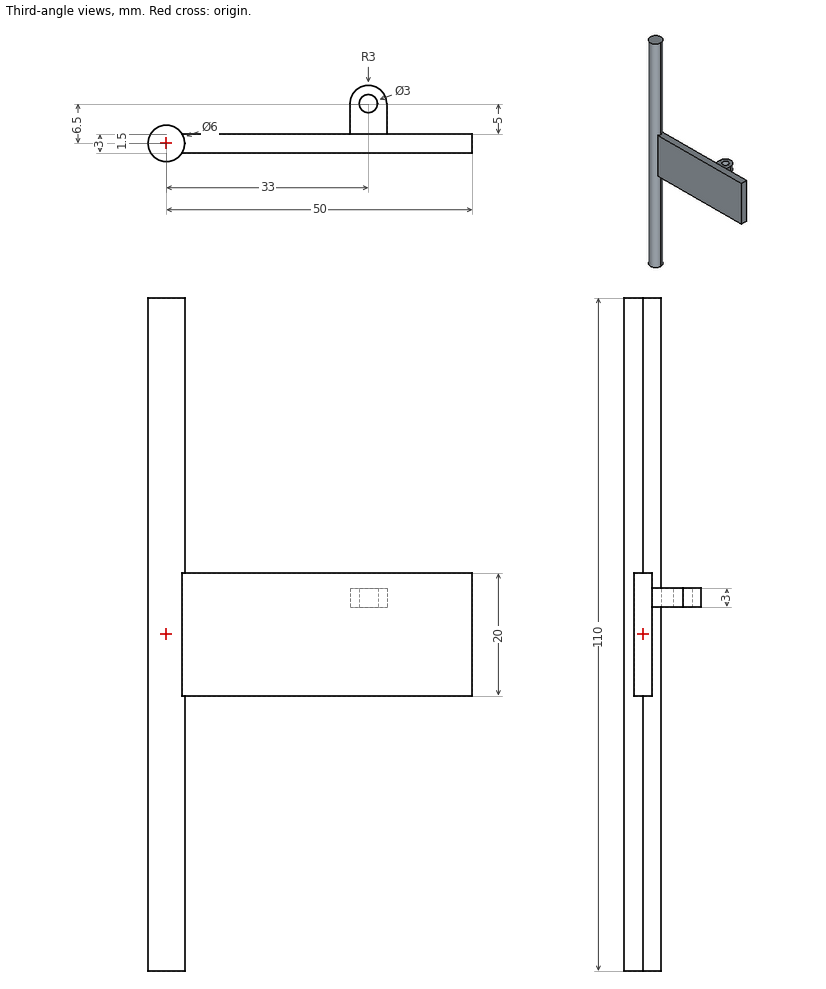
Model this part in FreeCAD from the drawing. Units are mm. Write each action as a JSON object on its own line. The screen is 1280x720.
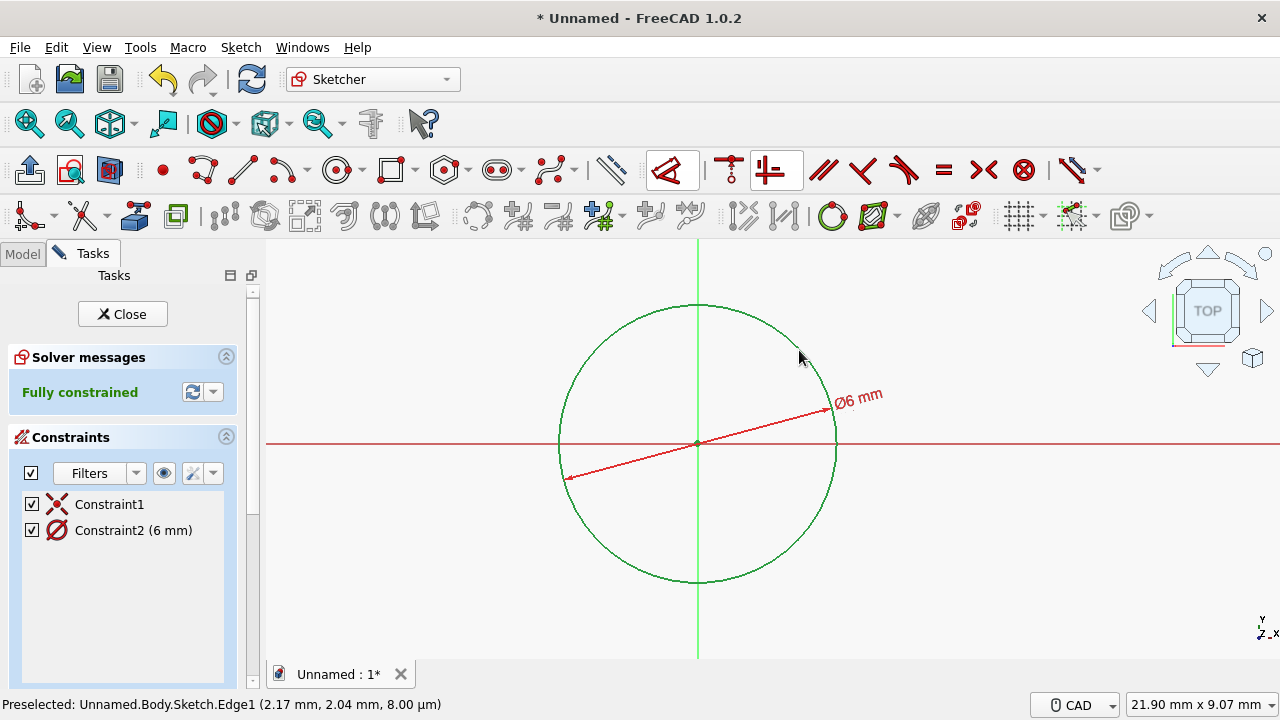
{"action": "left_click", "coordinate": [123, 314]}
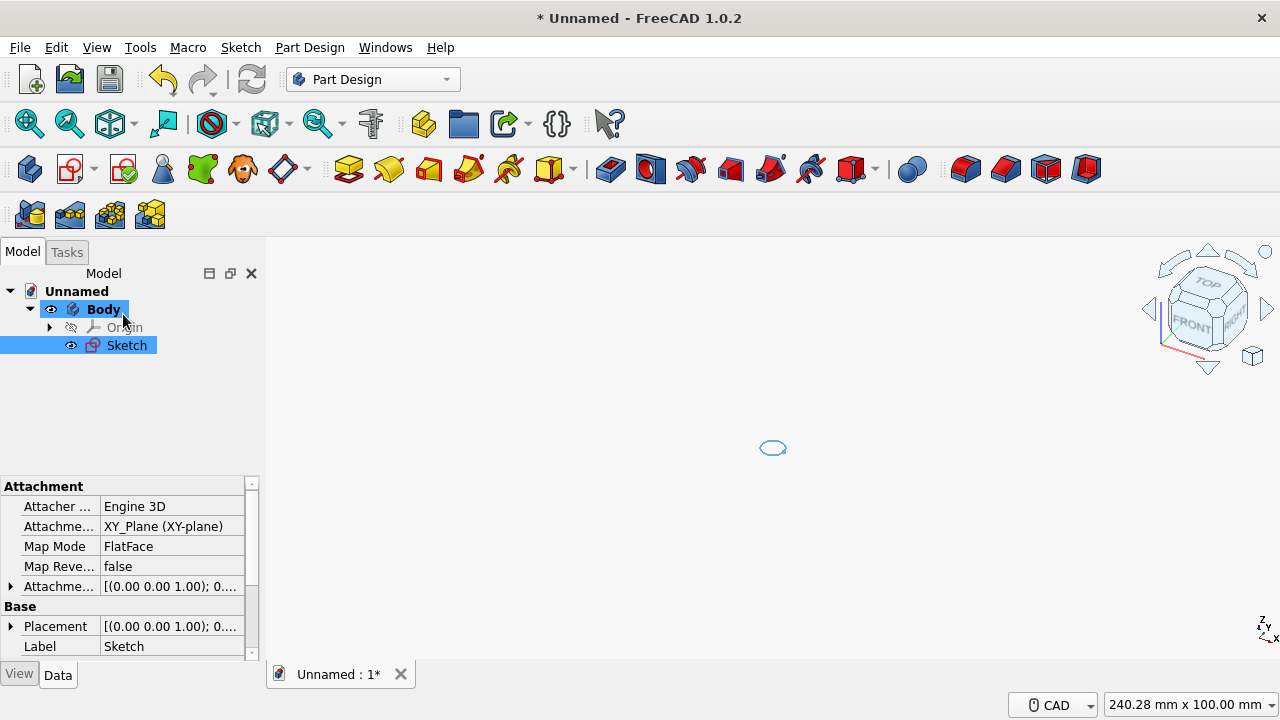
{"action": "left_click", "coordinate": [350, 170]}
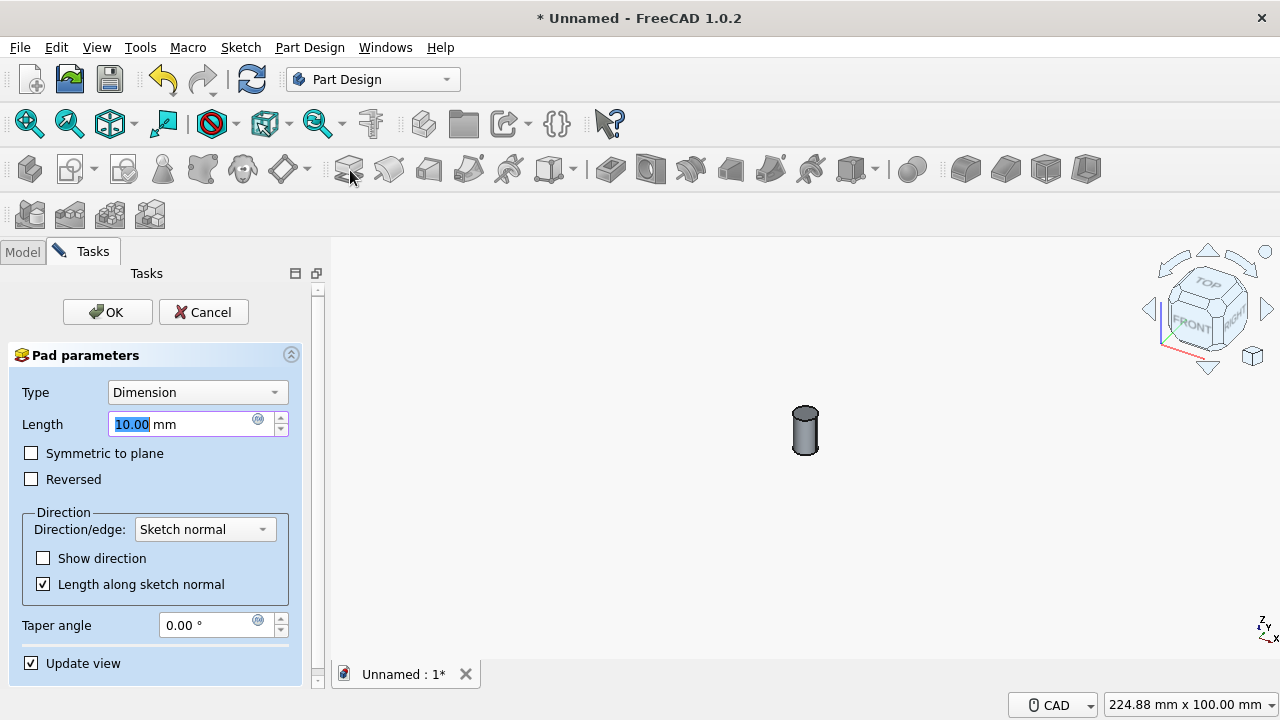
{"action": "type", "text": "110"}
{"action": "key", "text": "Tab"}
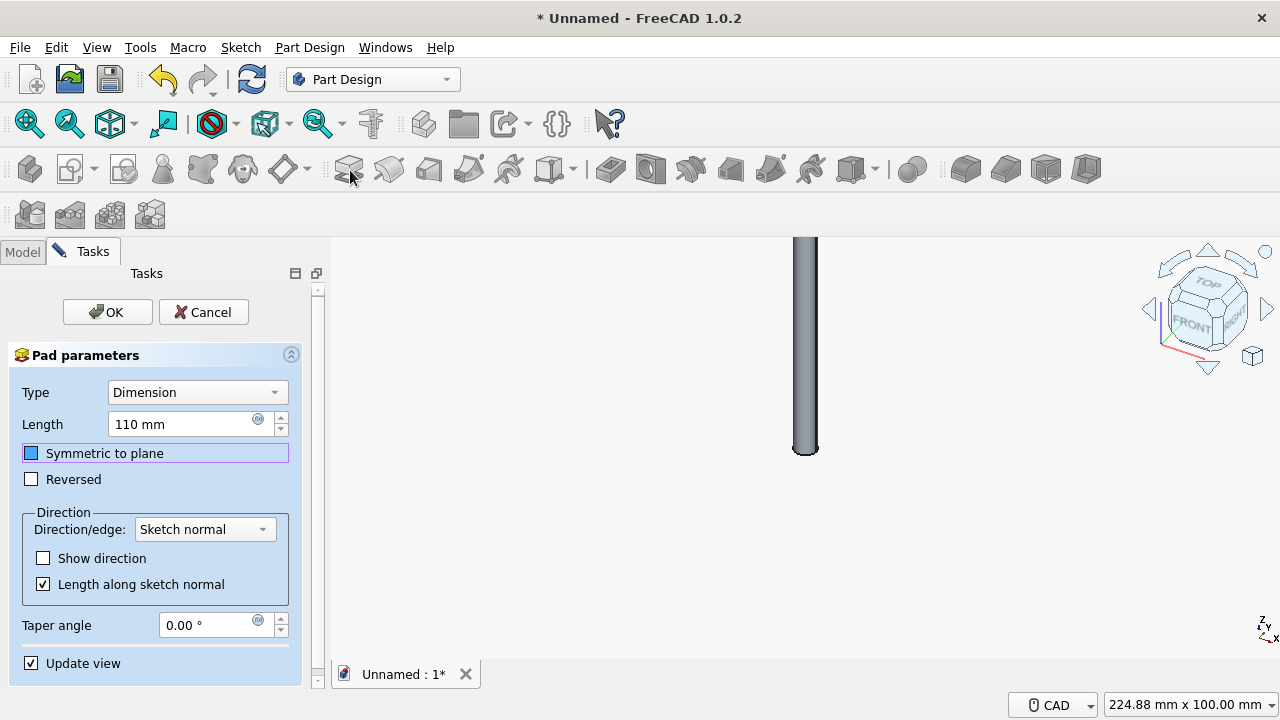
{"action": "left_click", "coordinate": [30, 453]}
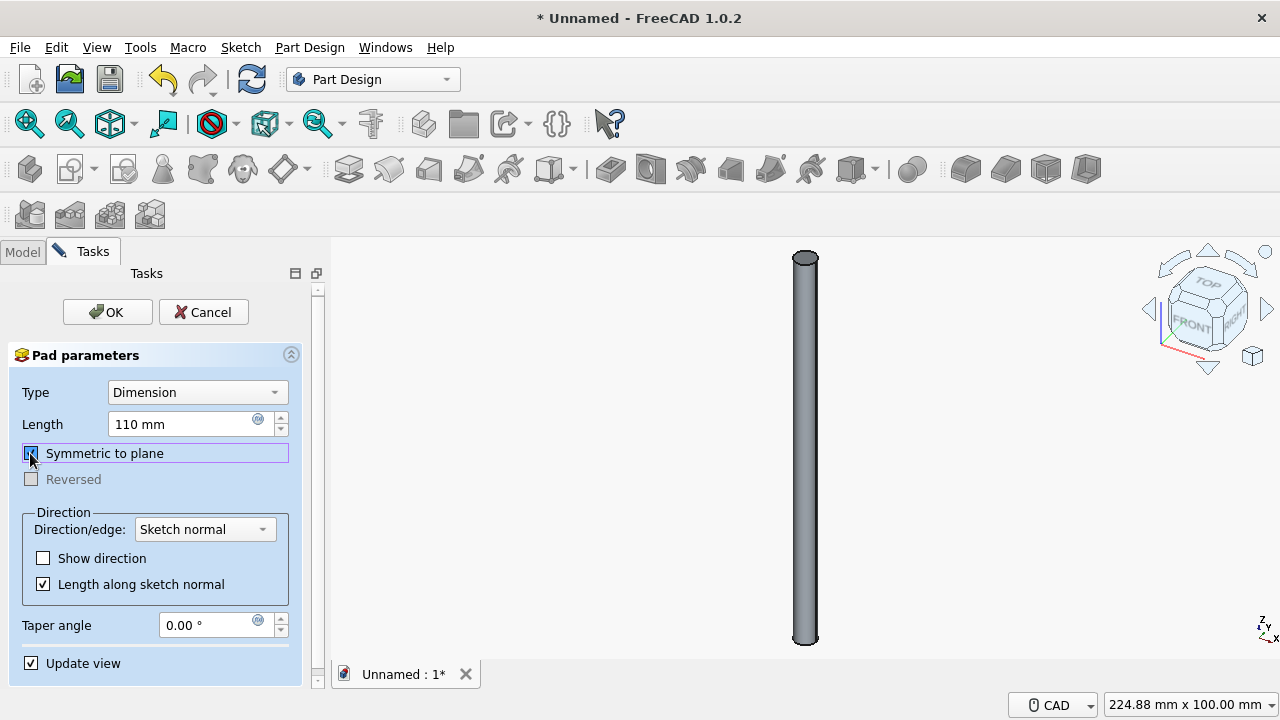
{"action": "left_click", "coordinate": [108, 312]}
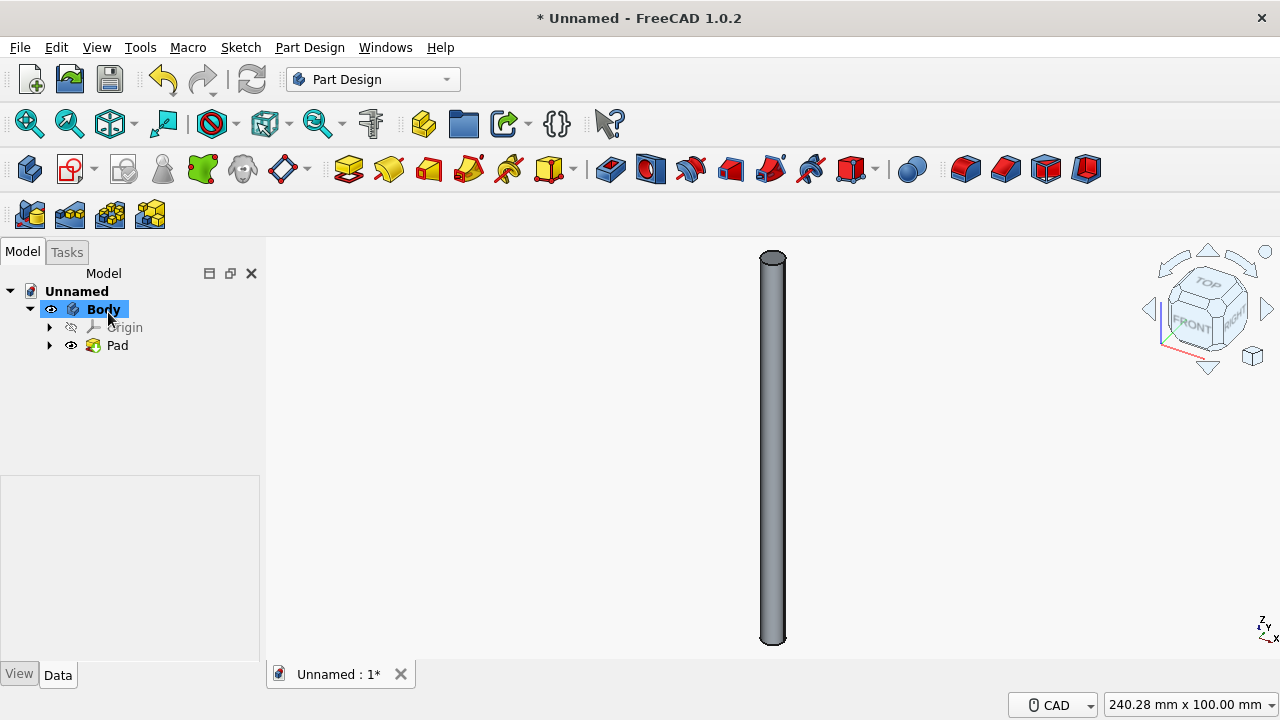
{"action": "left_click", "coordinate": [70, 170]}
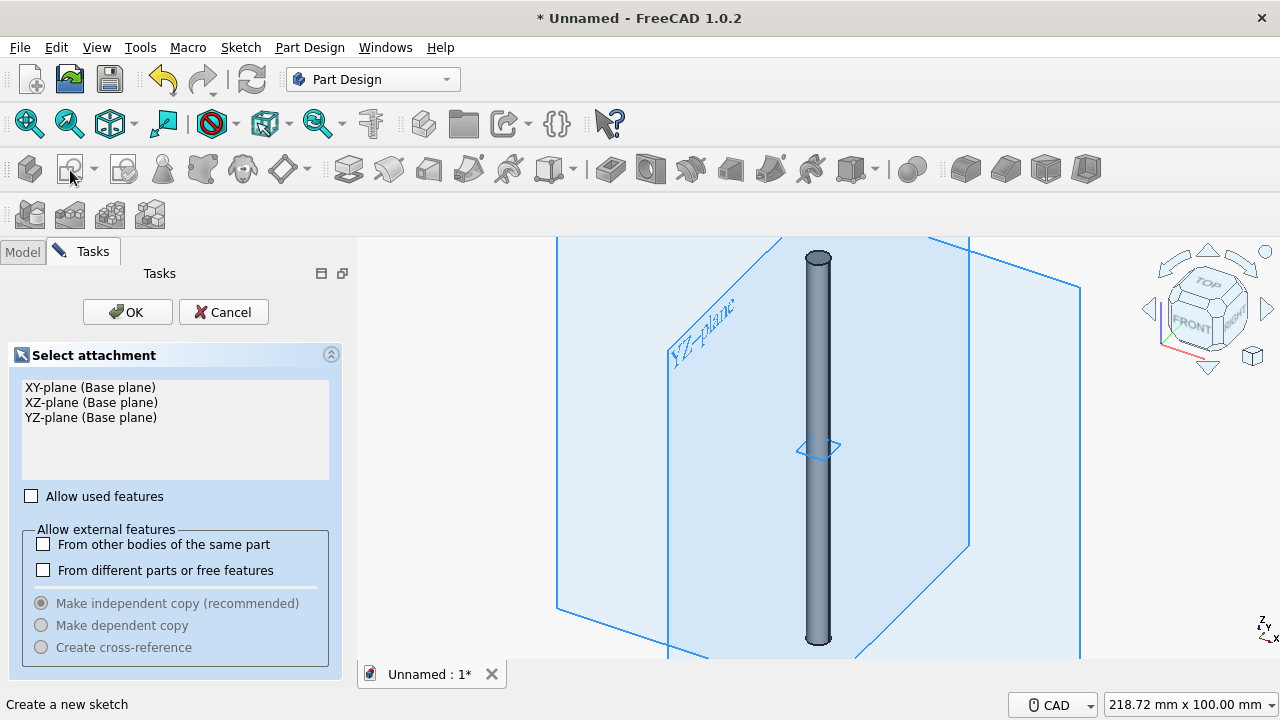
{"action": "left_click", "coordinate": [82, 388]}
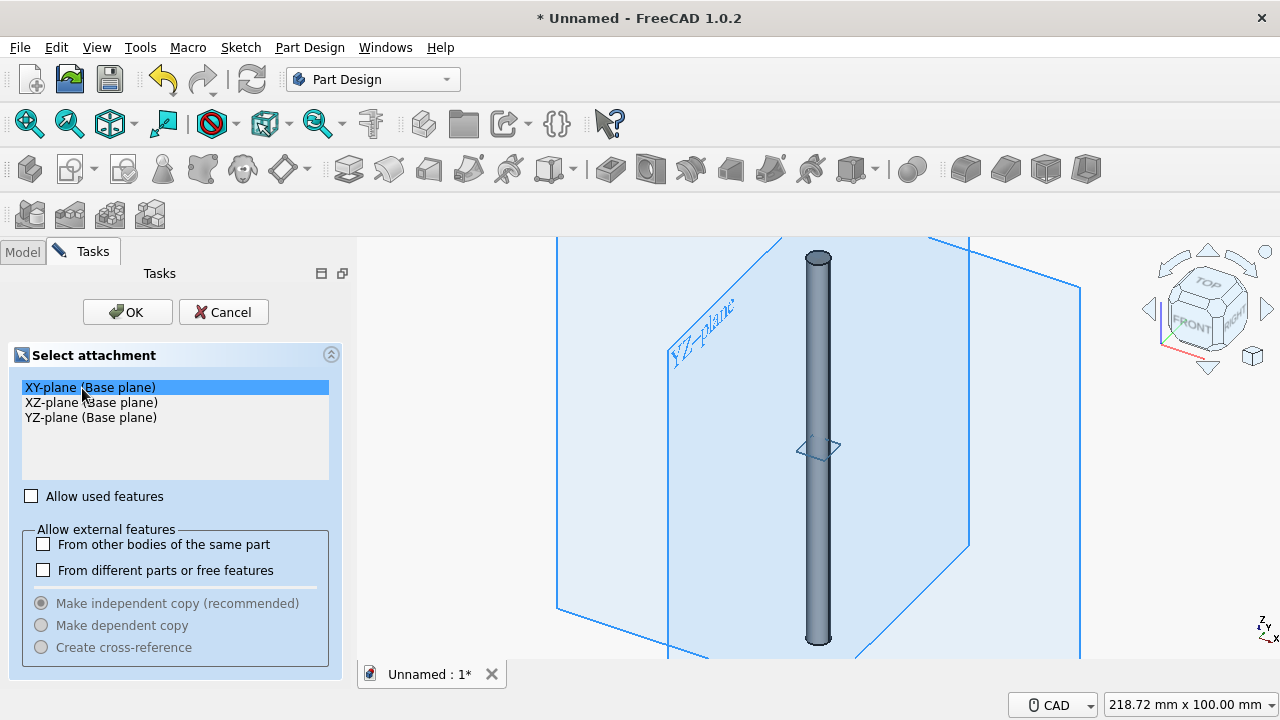
{"action": "left_click", "coordinate": [128, 312]}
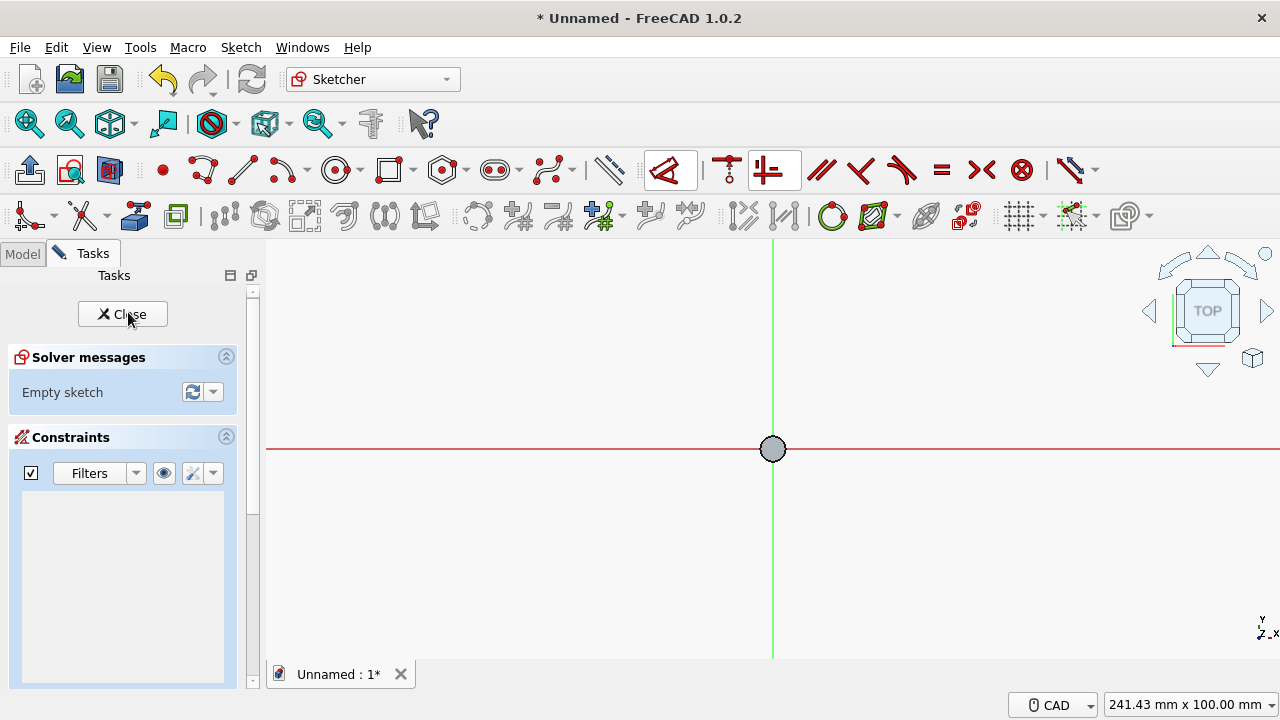
{"action": "left_click", "coordinate": [110, 170]}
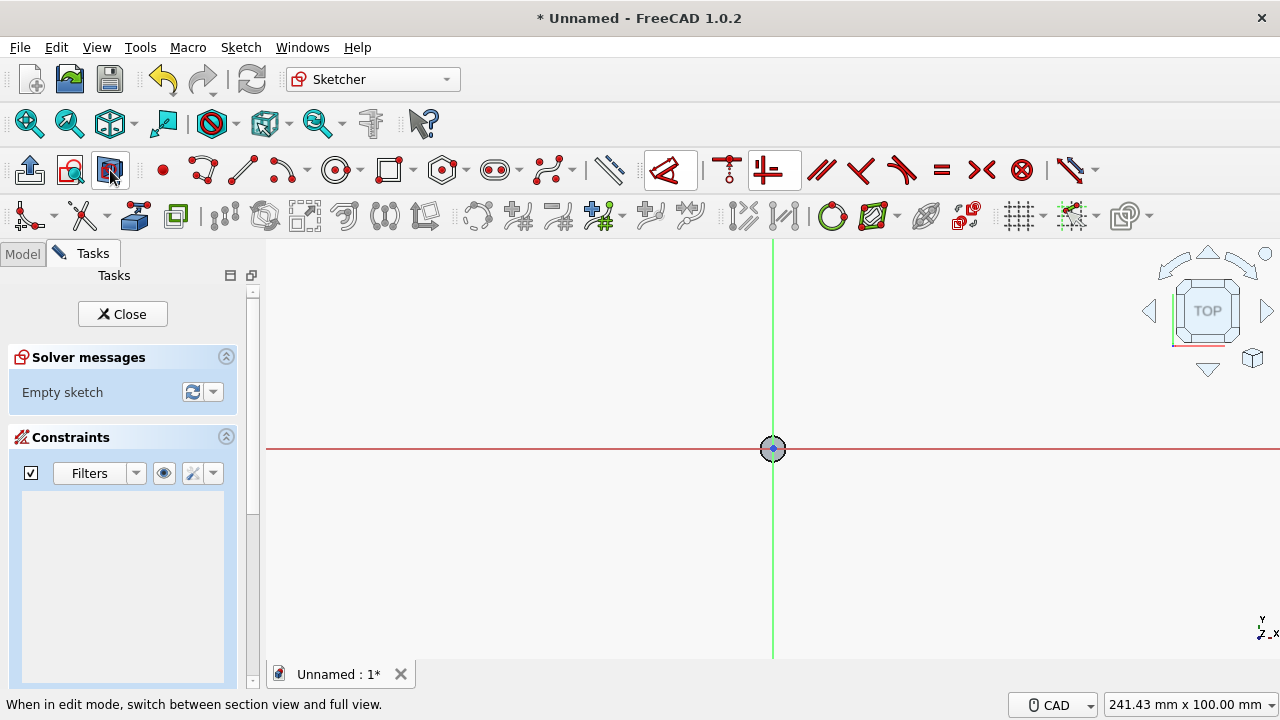
{"action": "scroll", "coordinate": [979, 449], "scroll_direction": "up", "scroll_amount": 5}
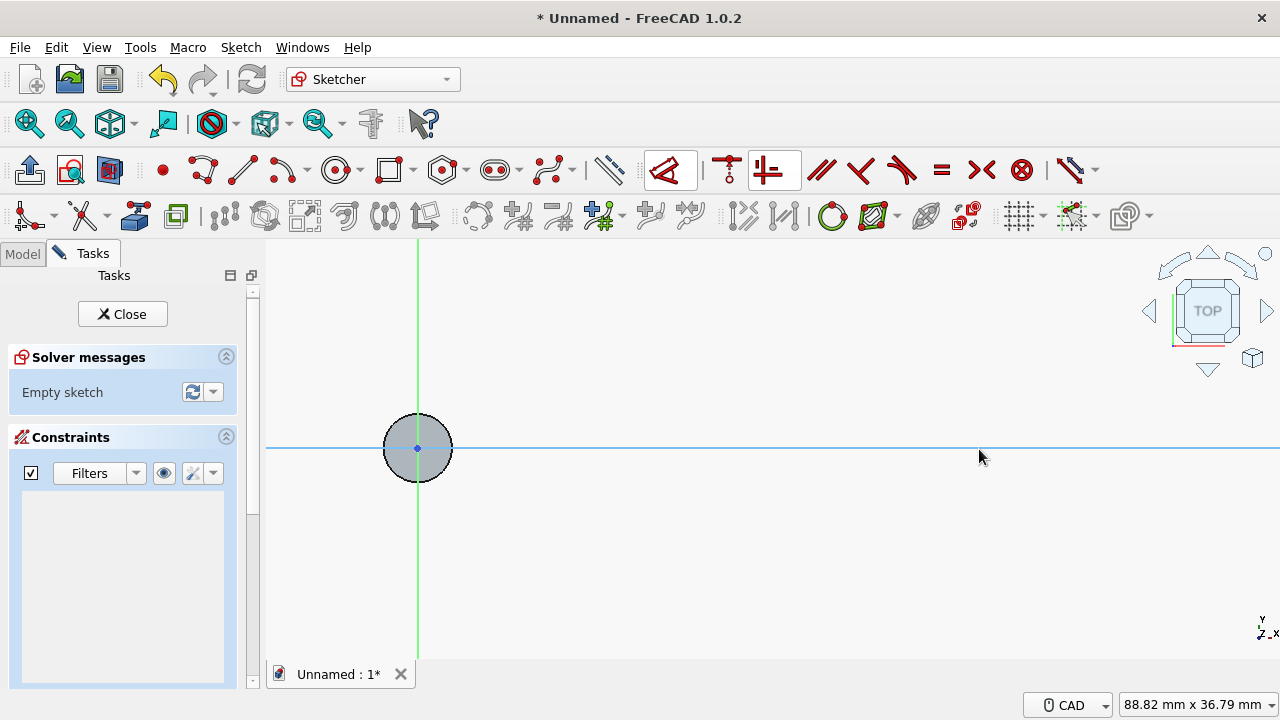
{"action": "left_click", "coordinate": [390, 170]}